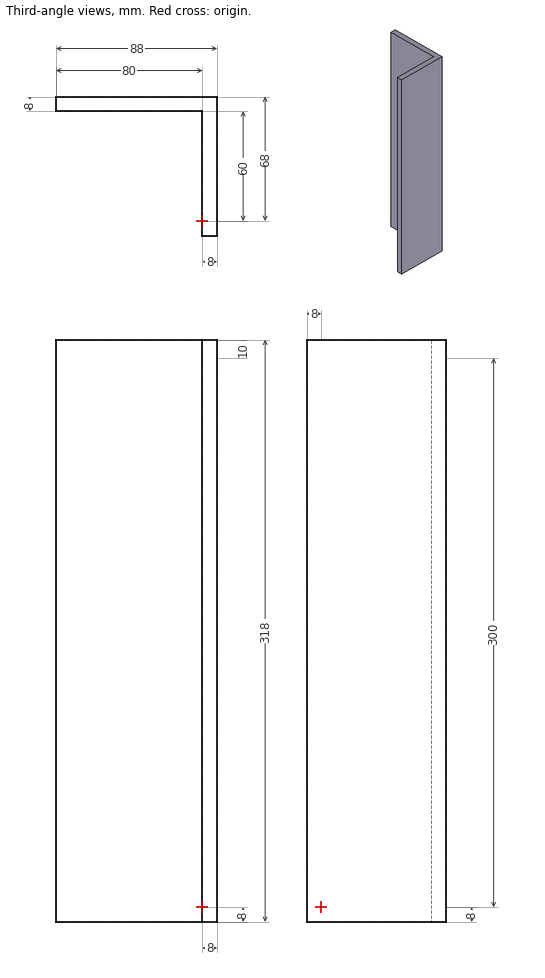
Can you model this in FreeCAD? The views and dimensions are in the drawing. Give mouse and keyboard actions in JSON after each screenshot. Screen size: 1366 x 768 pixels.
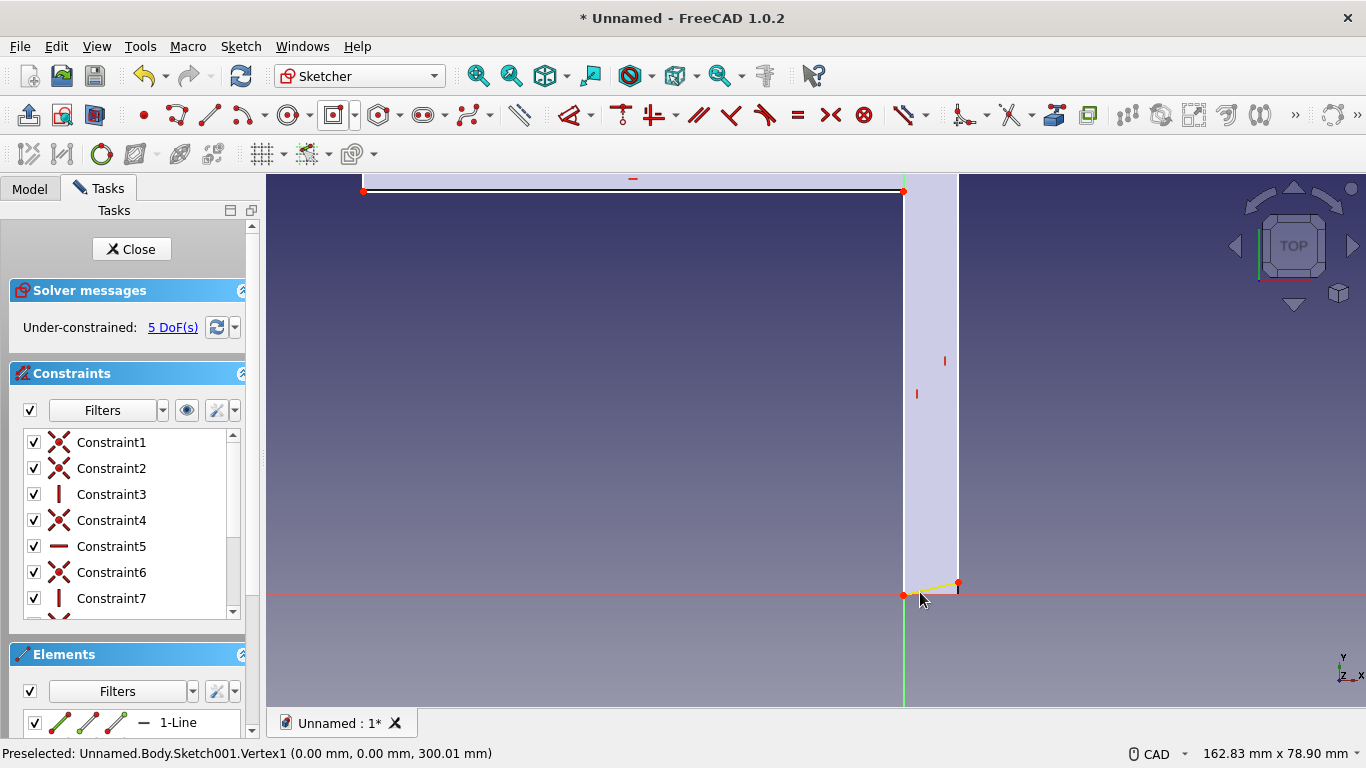
{"action": "left_click", "coordinate": [920, 592]}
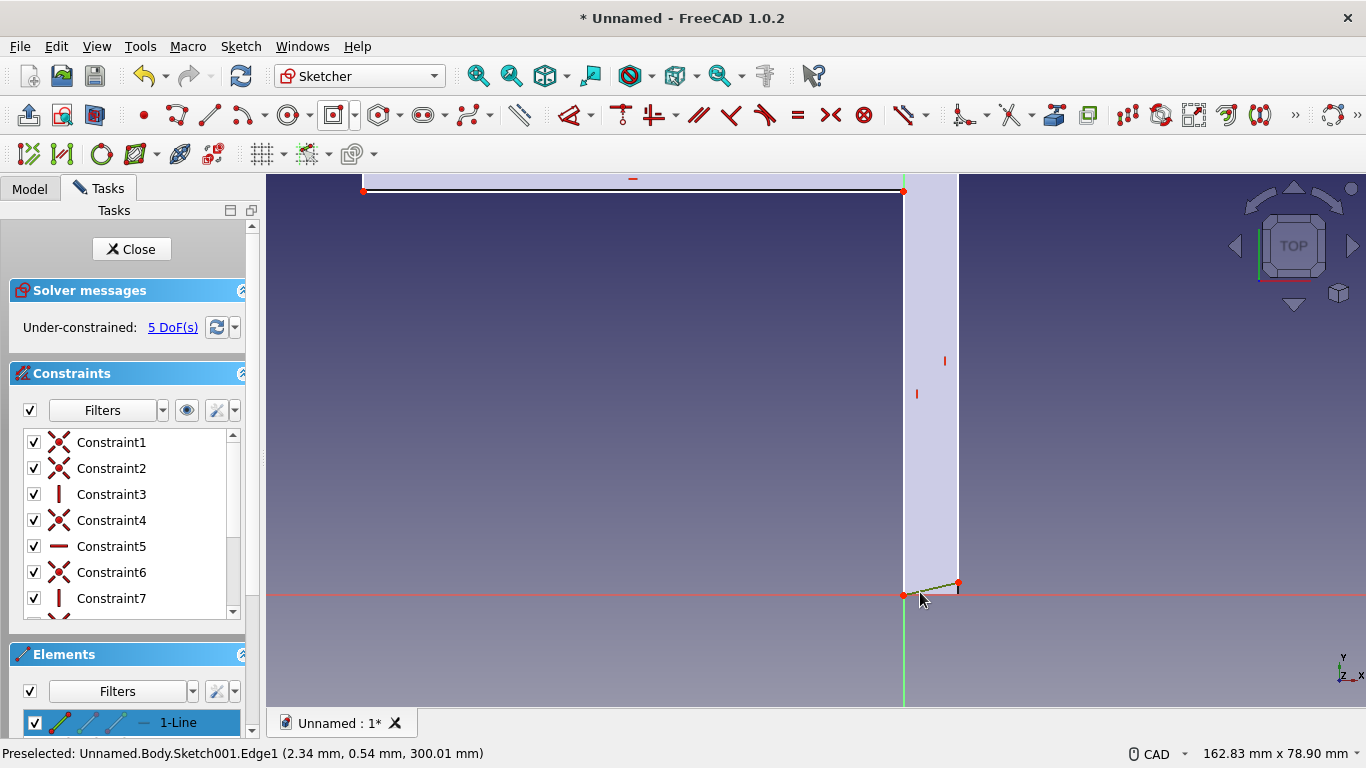
{"action": "left_click", "coordinate": [676, 116]}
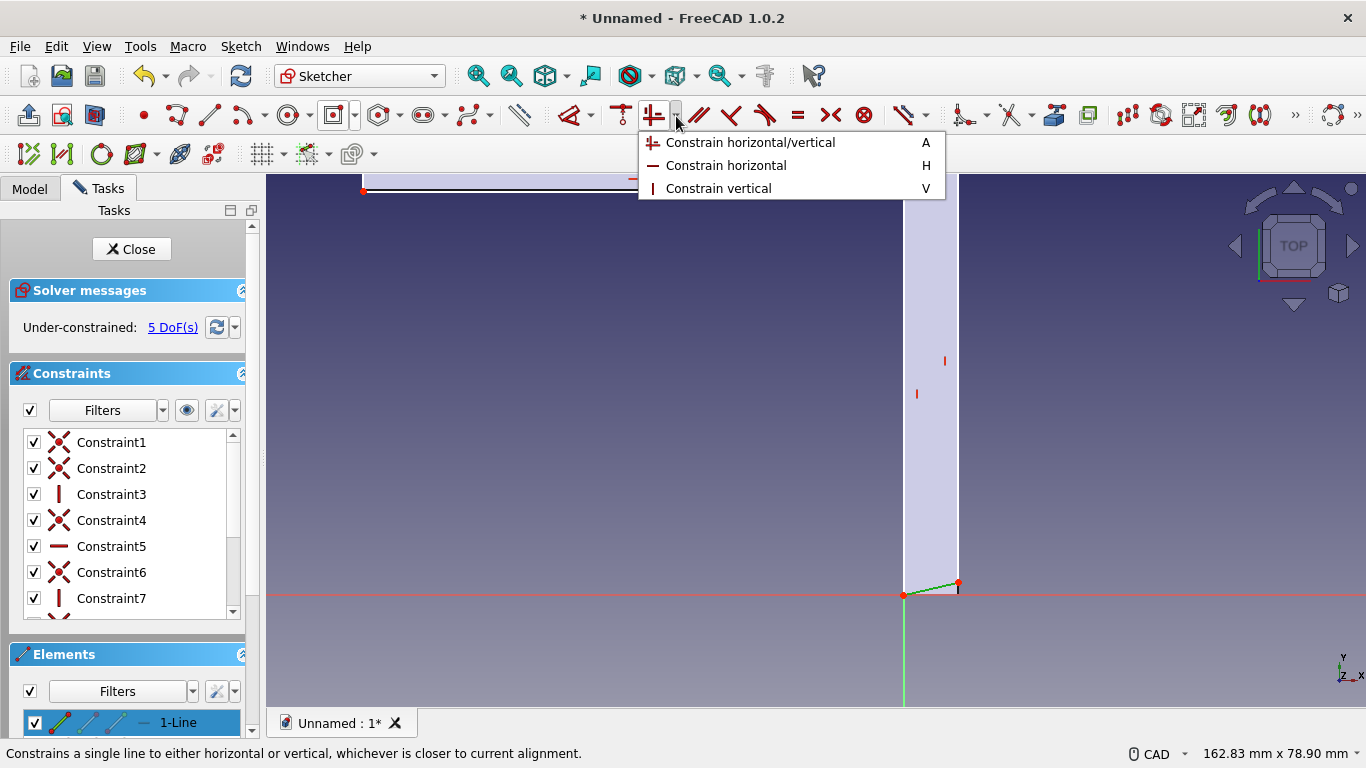
{"action": "left_click", "coordinate": [792, 166]}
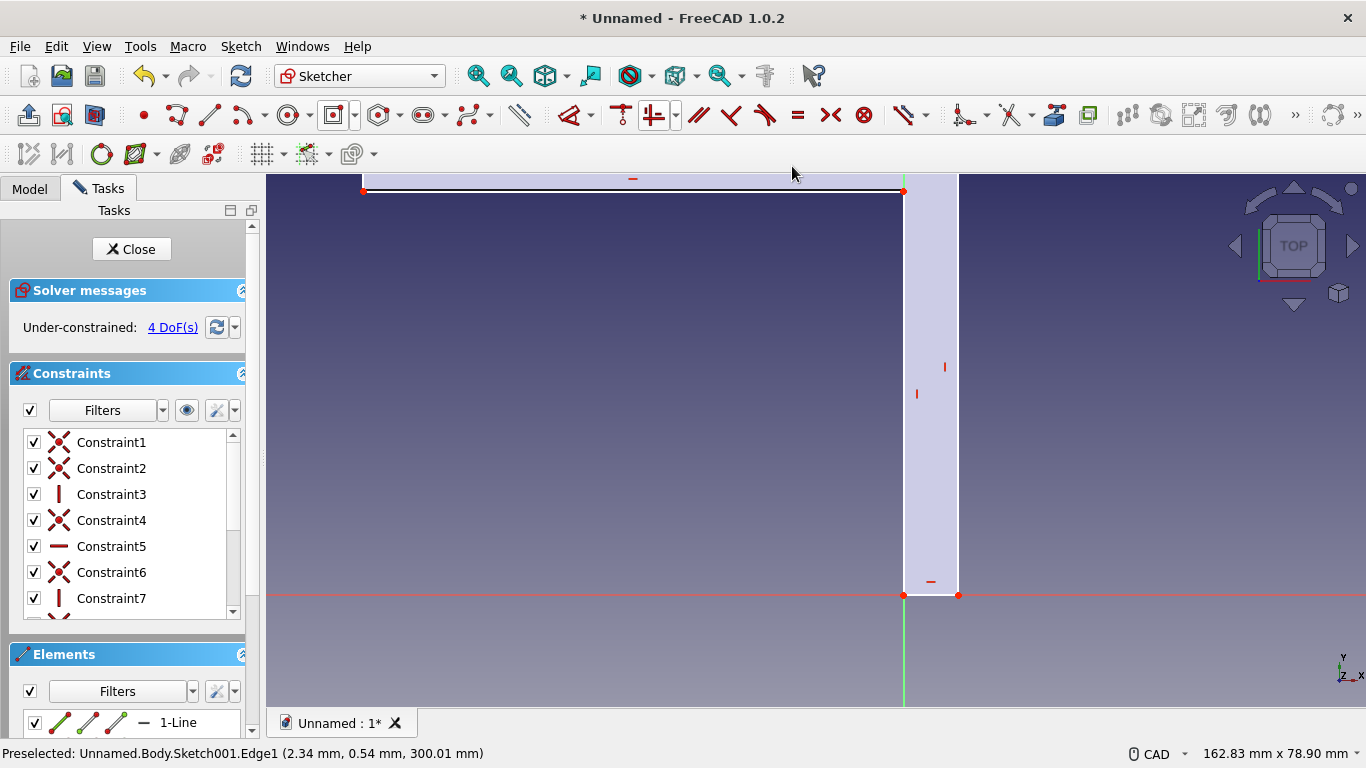
{"action": "left_click", "coordinate": [568, 116]}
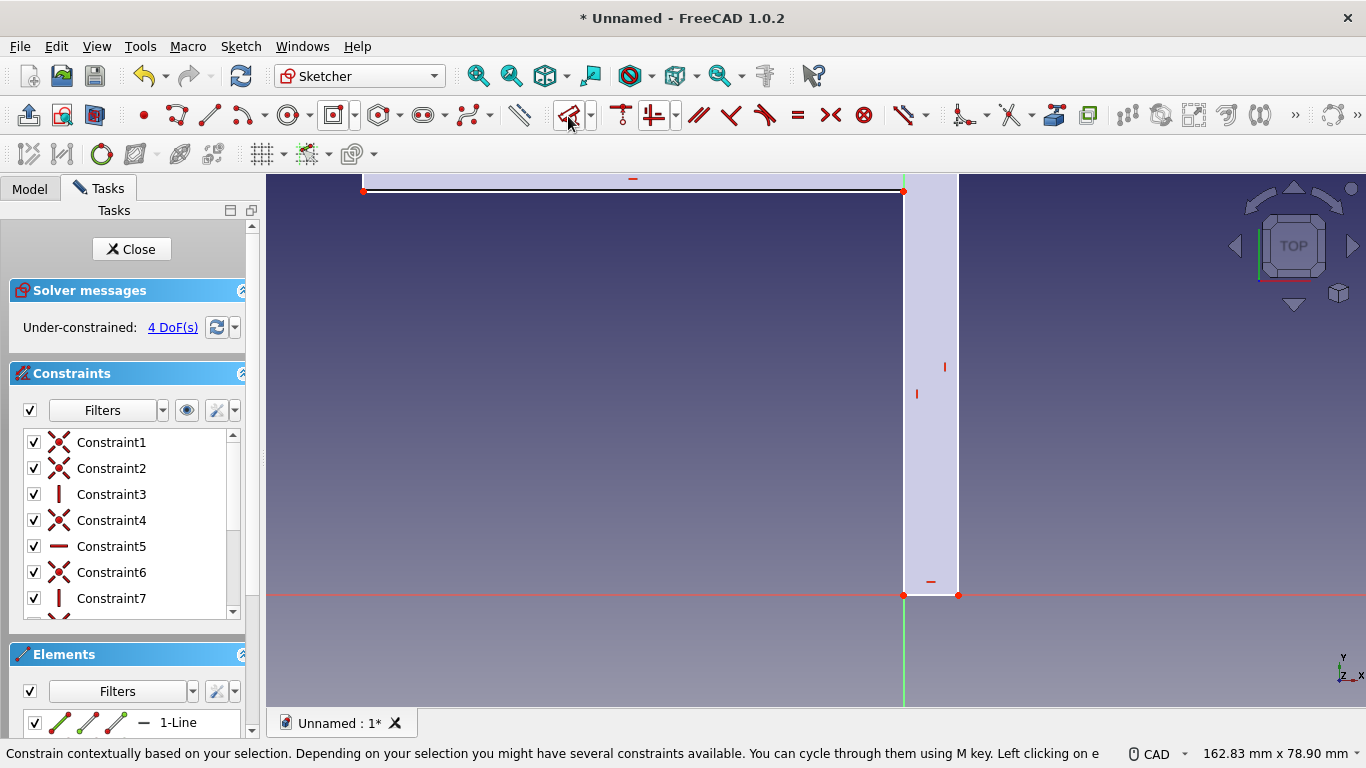
{"action": "left_click", "coordinate": [920, 595]}
{"action": "left_click", "coordinate": [931, 629]}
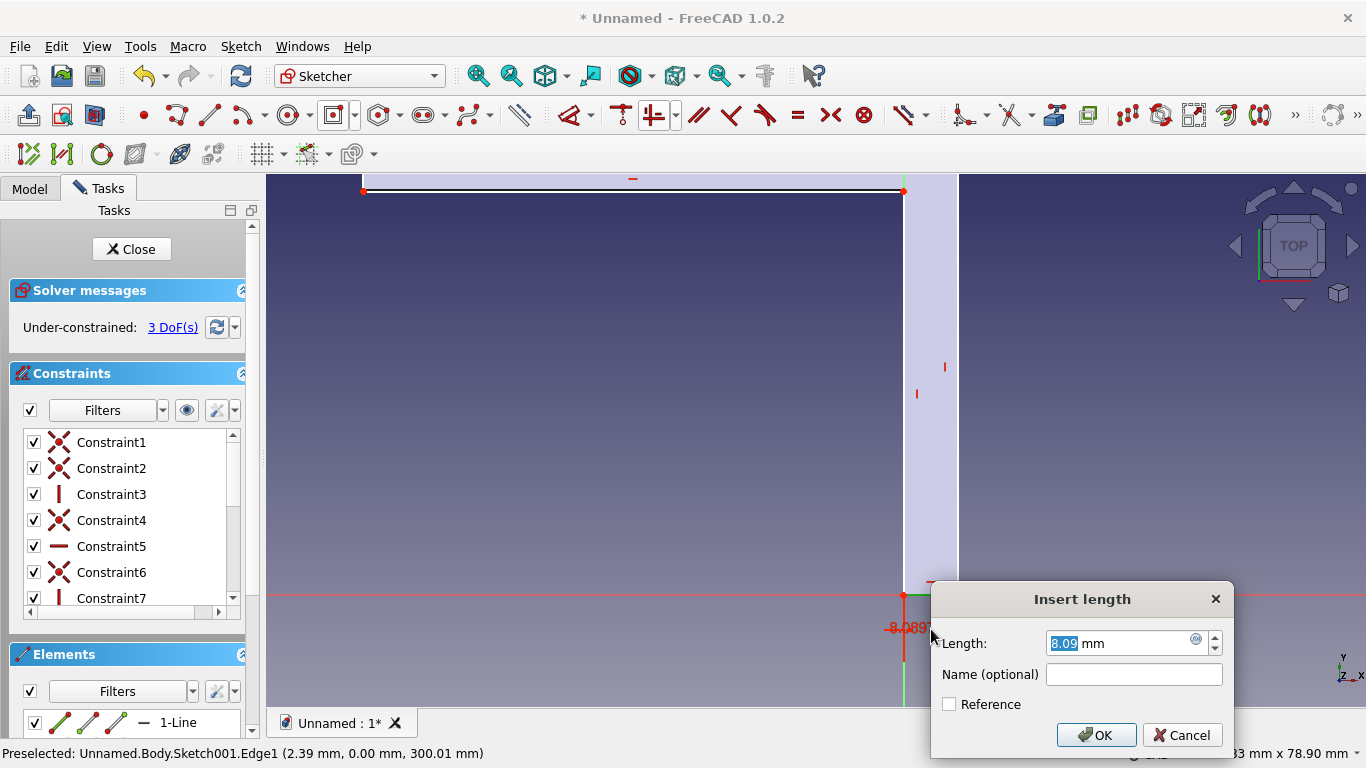
{"action": "type", "text": "8"}
{"action": "key", "text": "Return"}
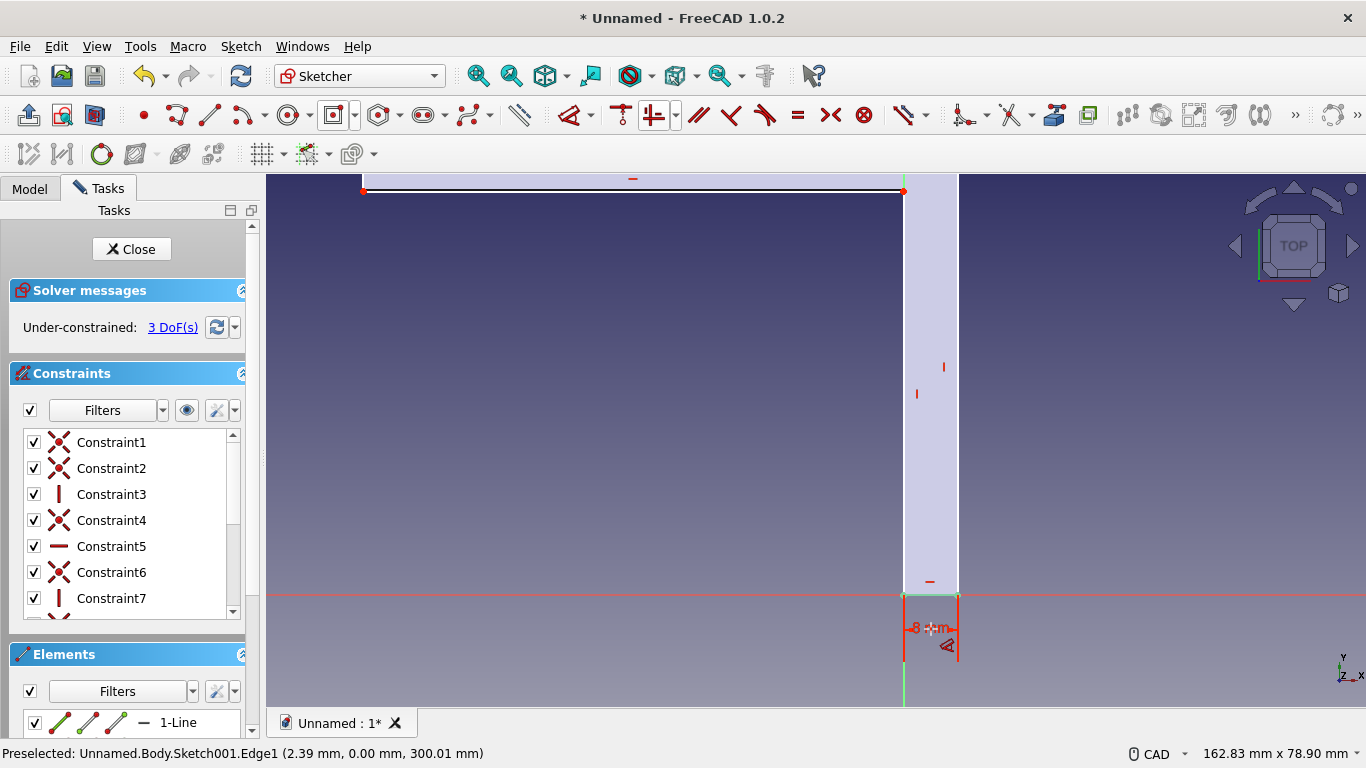
{"action": "scroll", "coordinate": [924, 593], "scroll_direction": "down", "scroll_amount": 2}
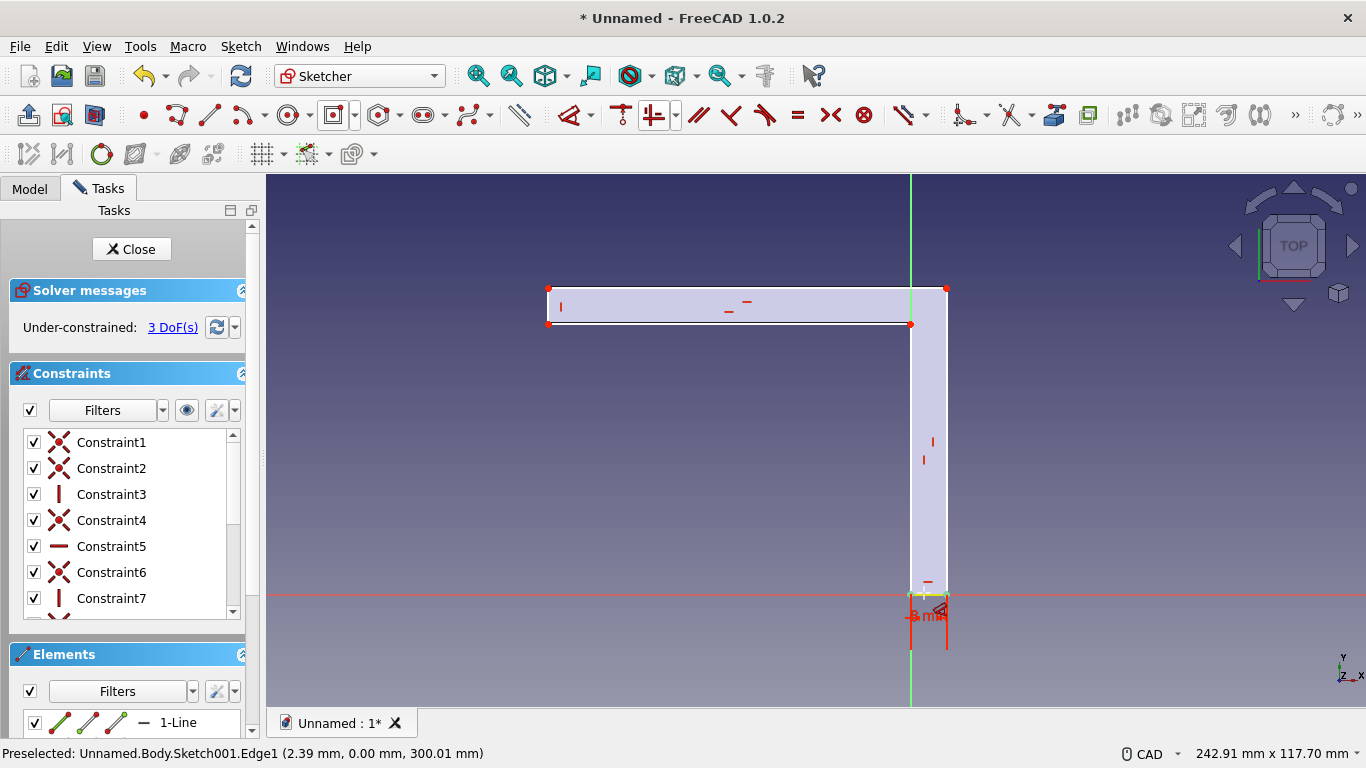
{"action": "scroll", "coordinate": [548, 299], "scroll_direction": "up", "scroll_amount": 2}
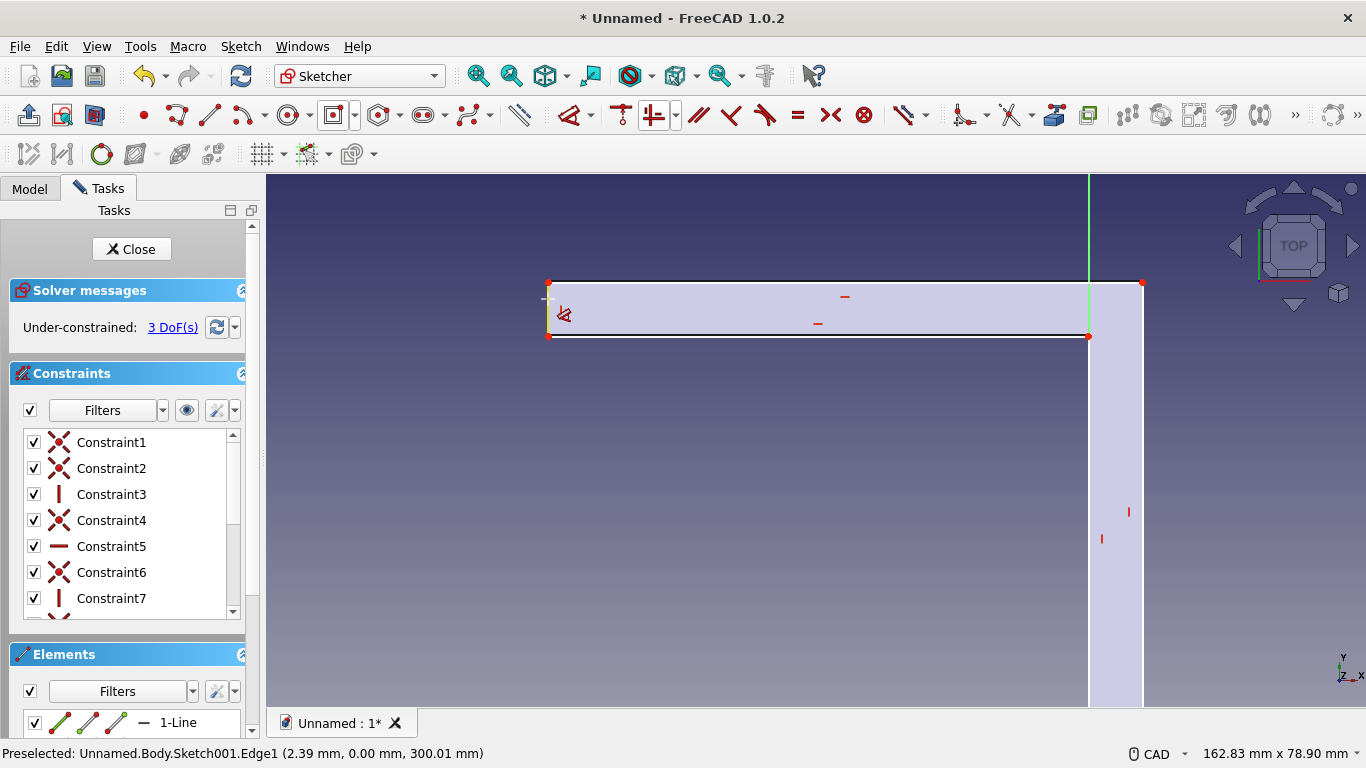
{"action": "left_click", "coordinate": [548, 299]}
{"action": "left_click", "coordinate": [514, 310]}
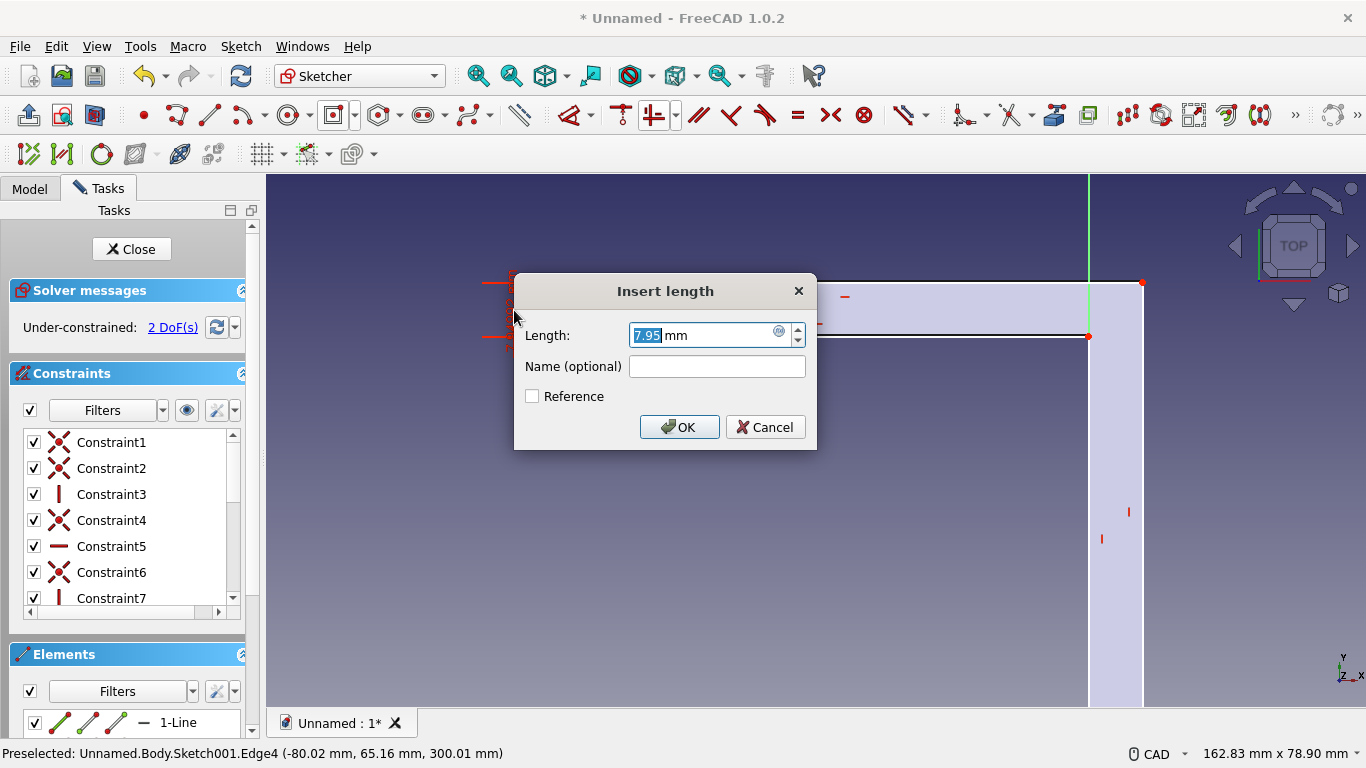
{"action": "type", "text": "8"}
{"action": "key", "text": "Return"}